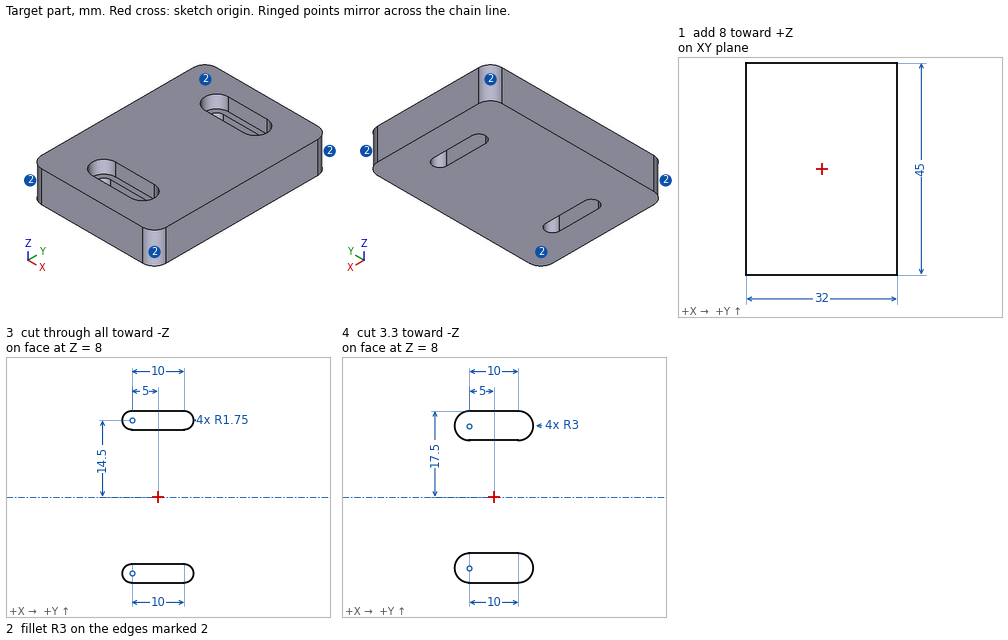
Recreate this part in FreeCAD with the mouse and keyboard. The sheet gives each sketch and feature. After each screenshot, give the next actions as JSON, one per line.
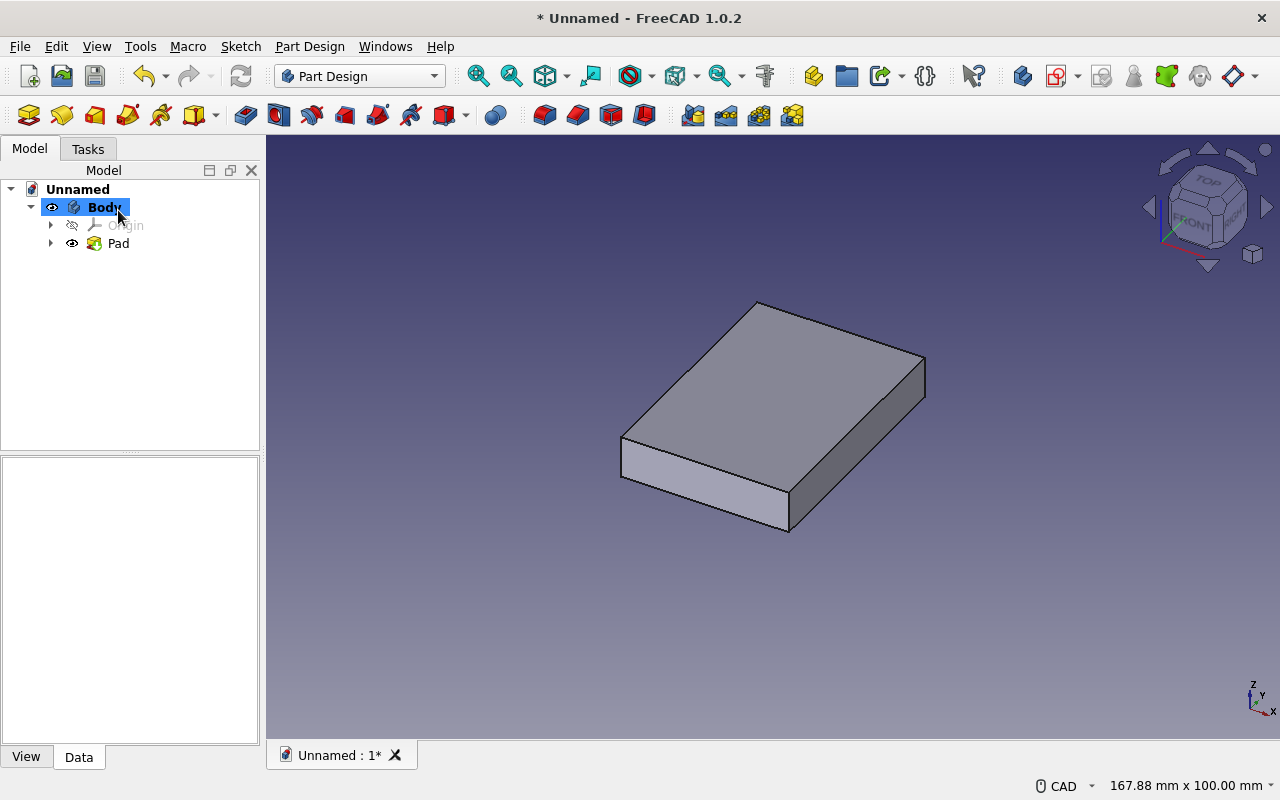
{"action": "left_click", "coordinate": [479, 76]}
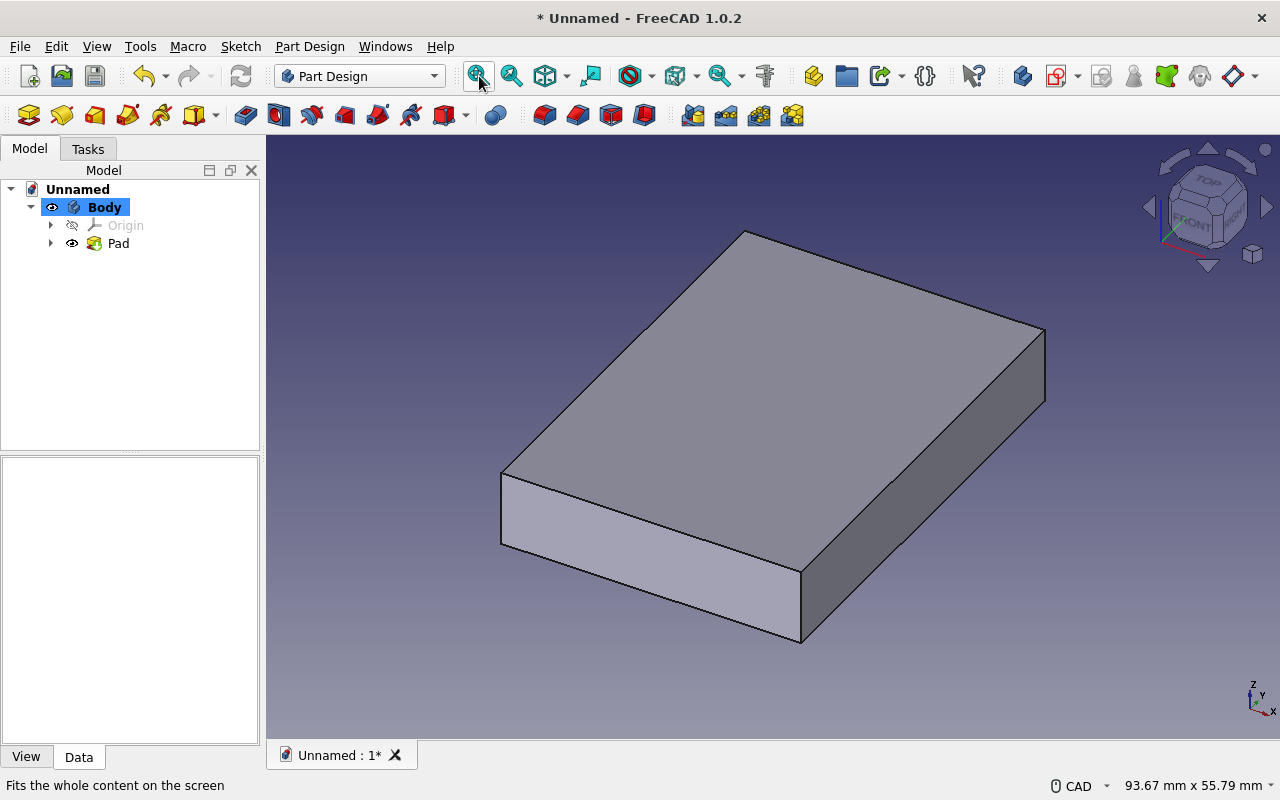
{"action": "left_click", "coordinate": [801, 607]}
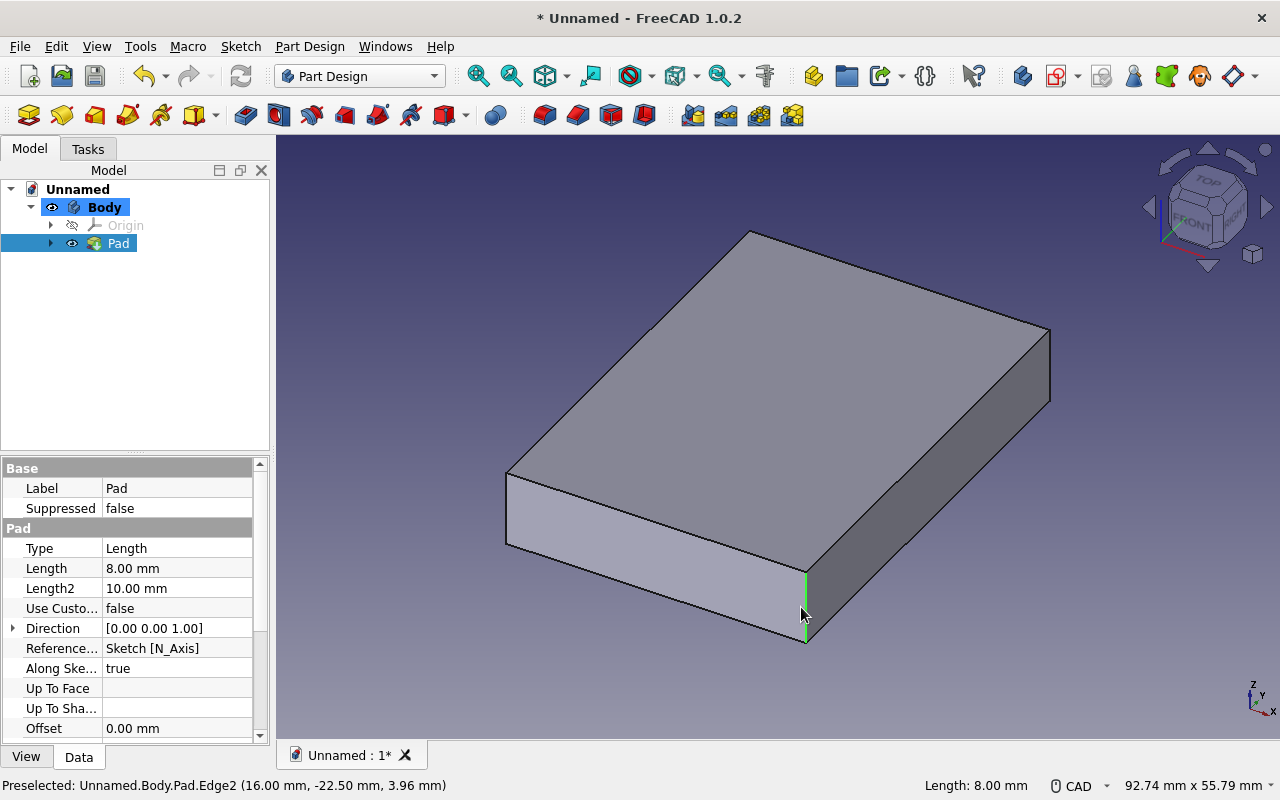
{"action": "key", "text": "0"}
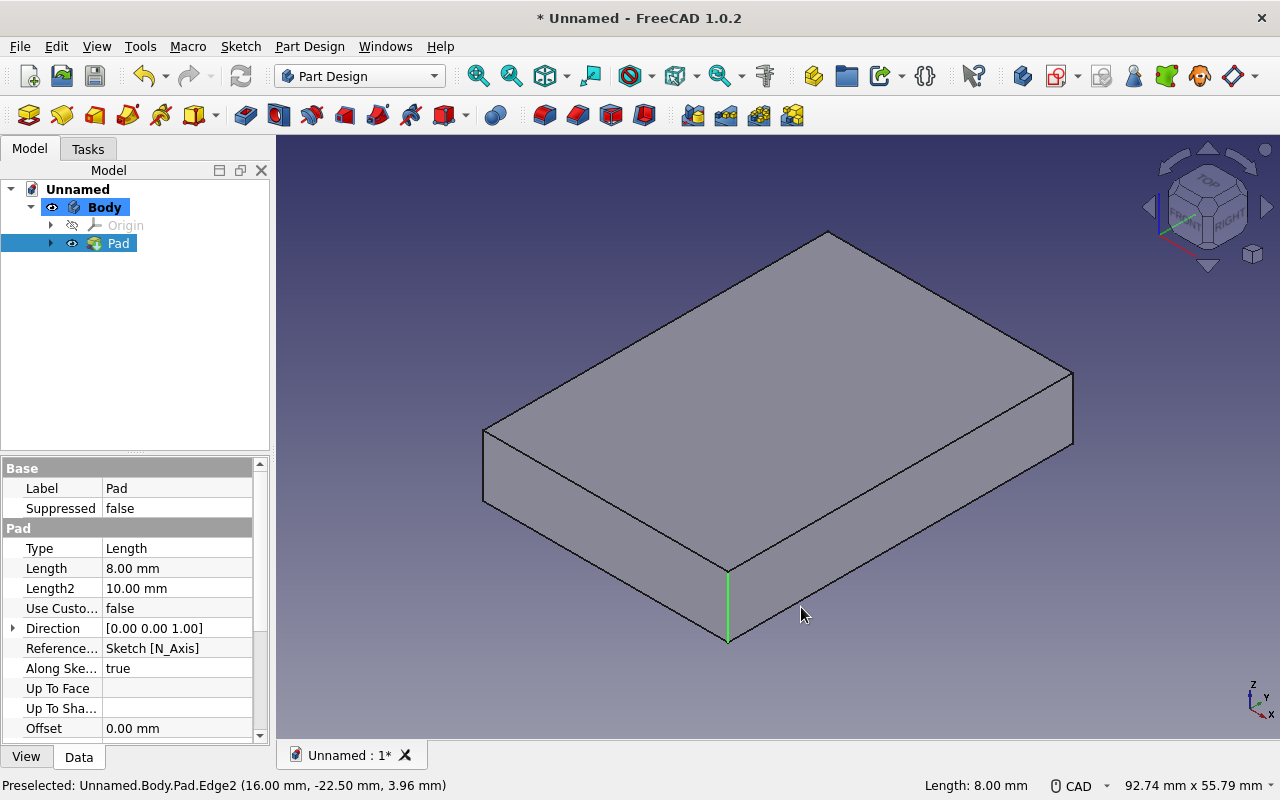
{"action": "key", "text": "2"}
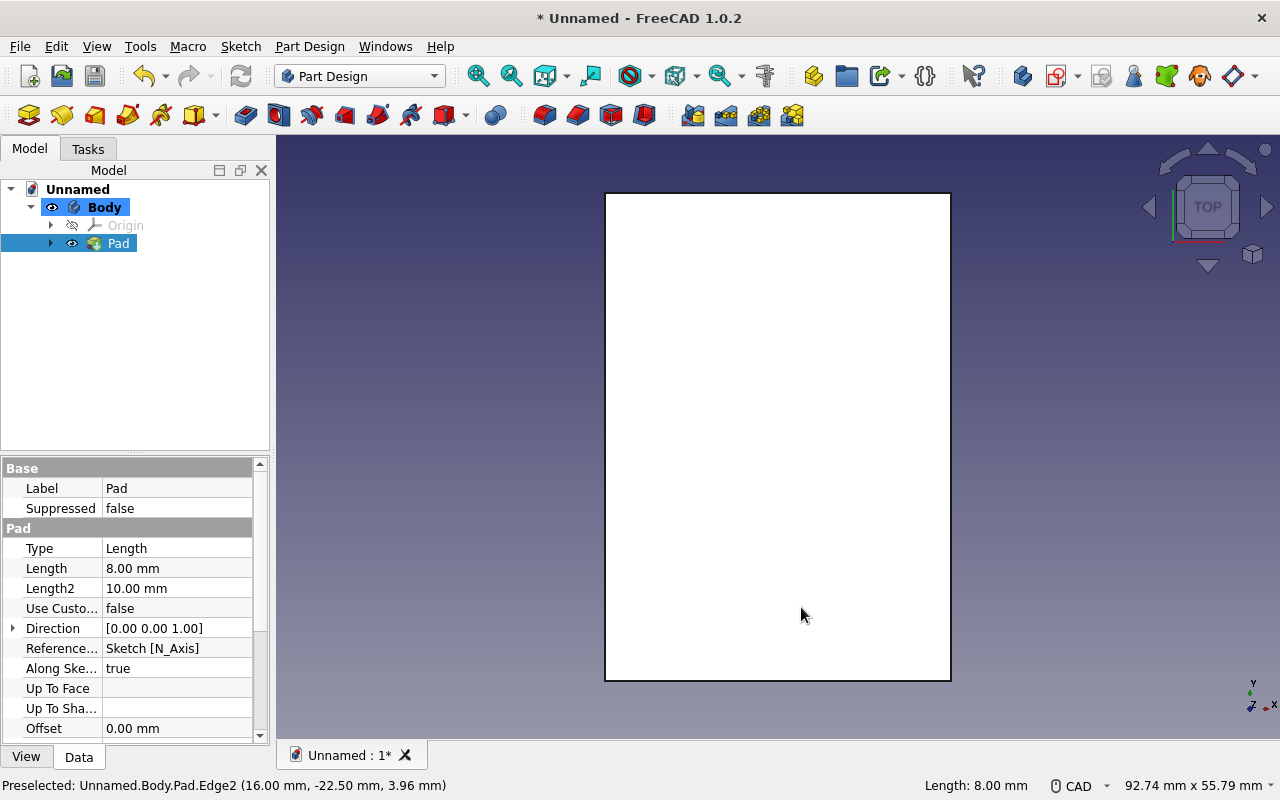
{"action": "key", "text": "1"}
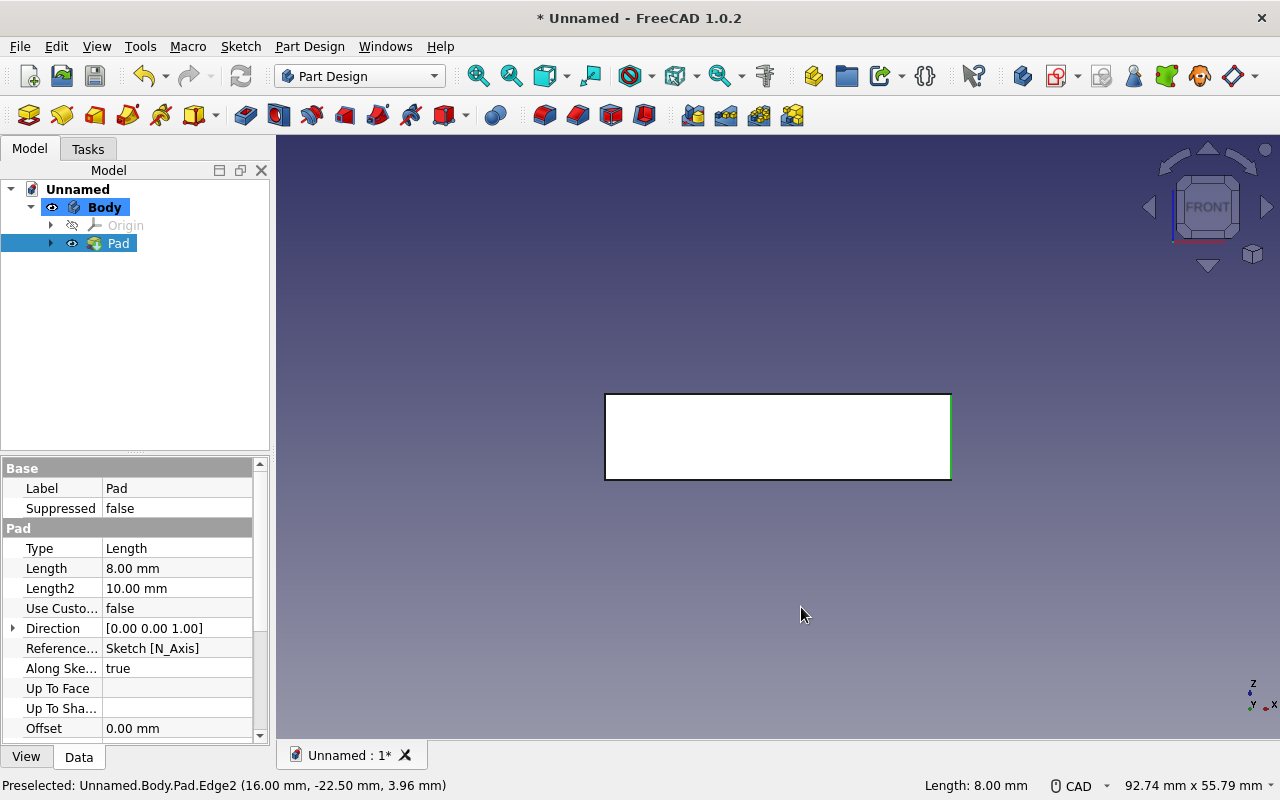
{"action": "left_click", "coordinate": [479, 76]}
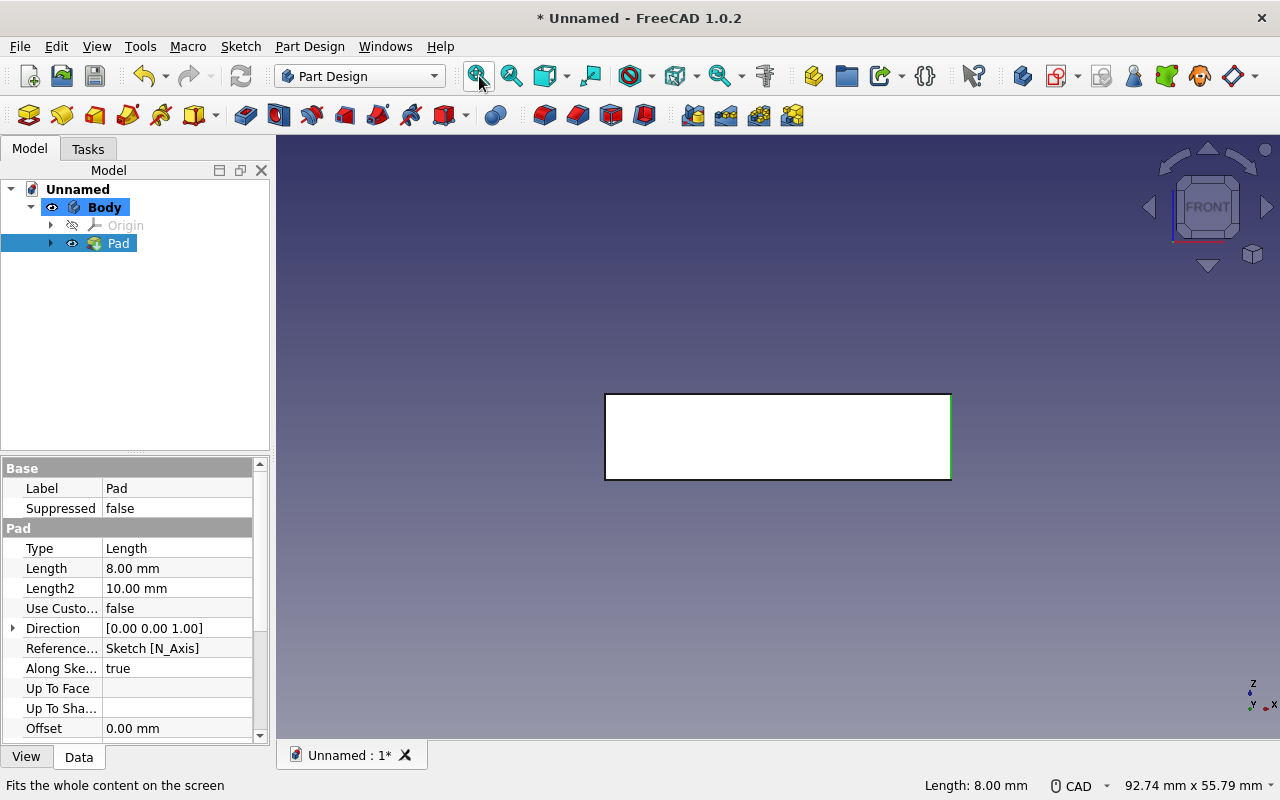
{"action": "left_click", "coordinate": [605, 436], "text": "ctrl"}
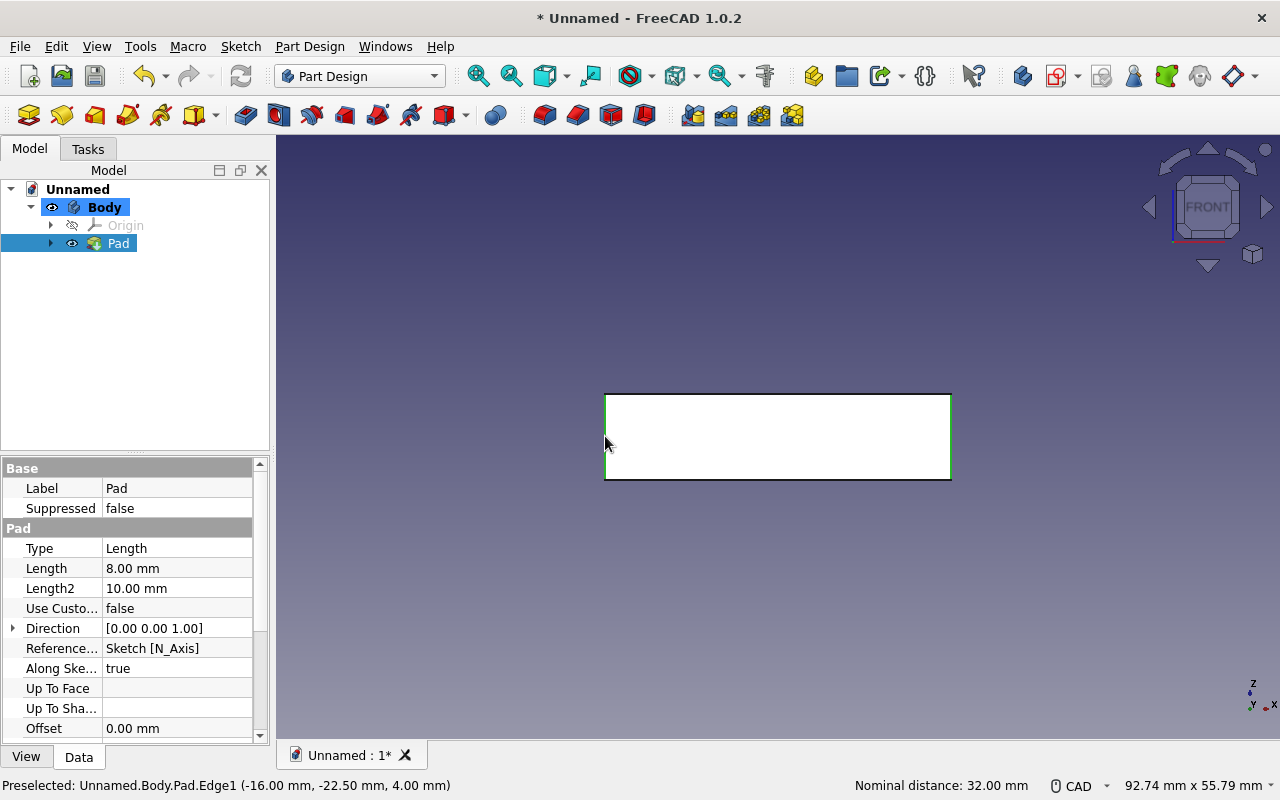
{"action": "key", "text": "3"}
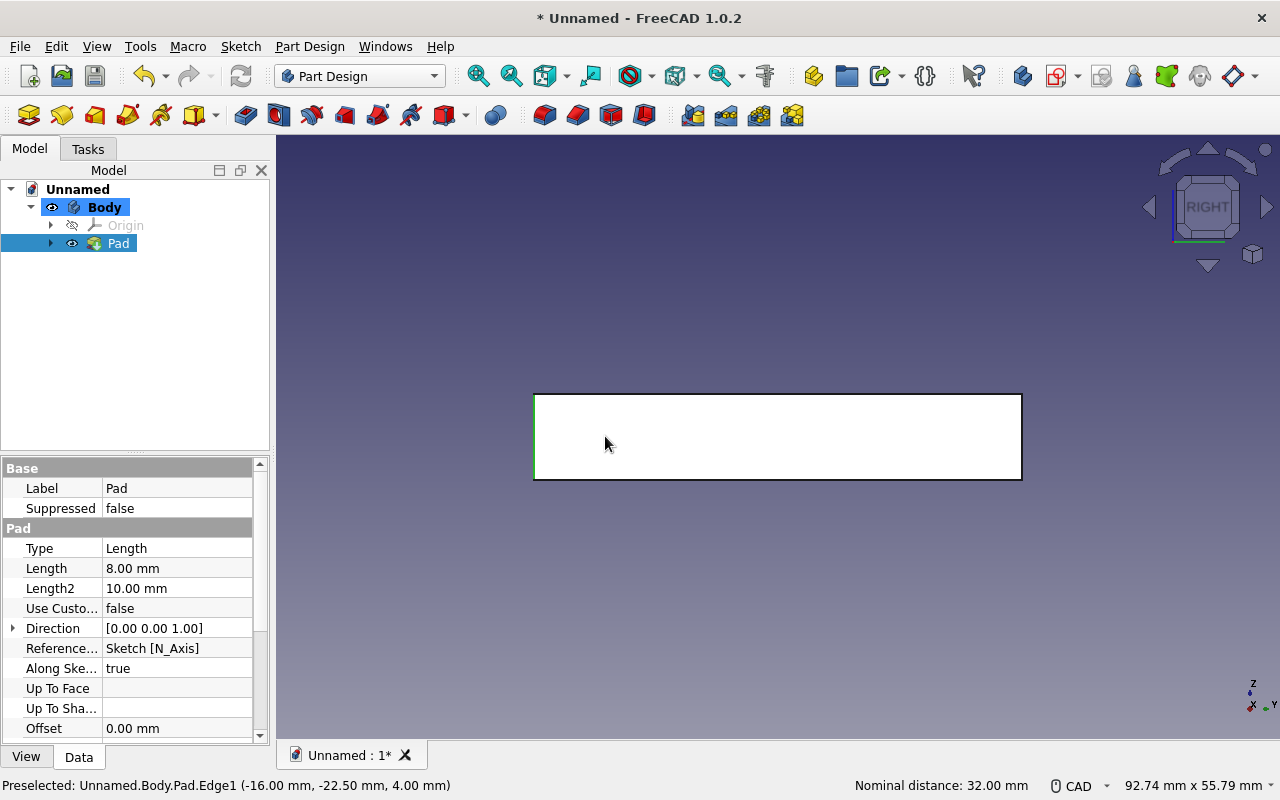
{"action": "left_click", "coordinate": [1022, 436], "text": "ctrl"}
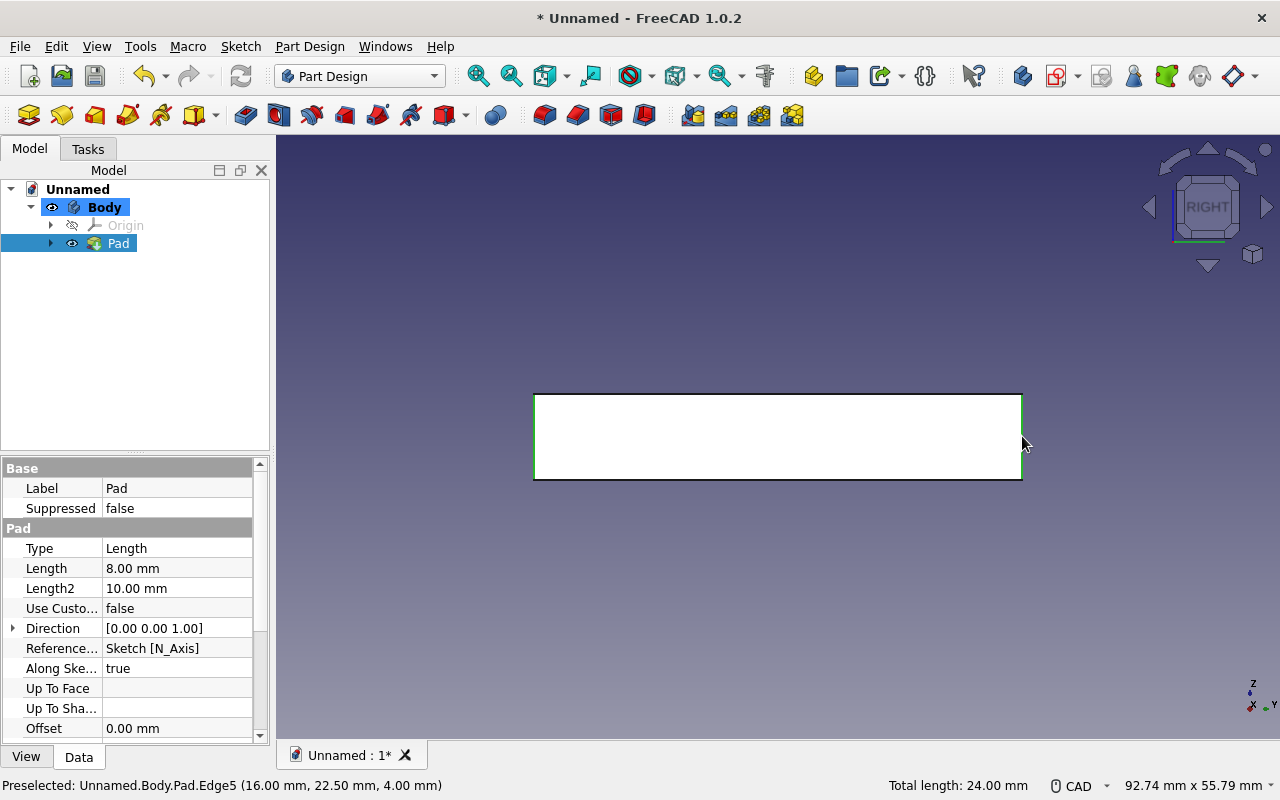
{"action": "key", "text": "5"}